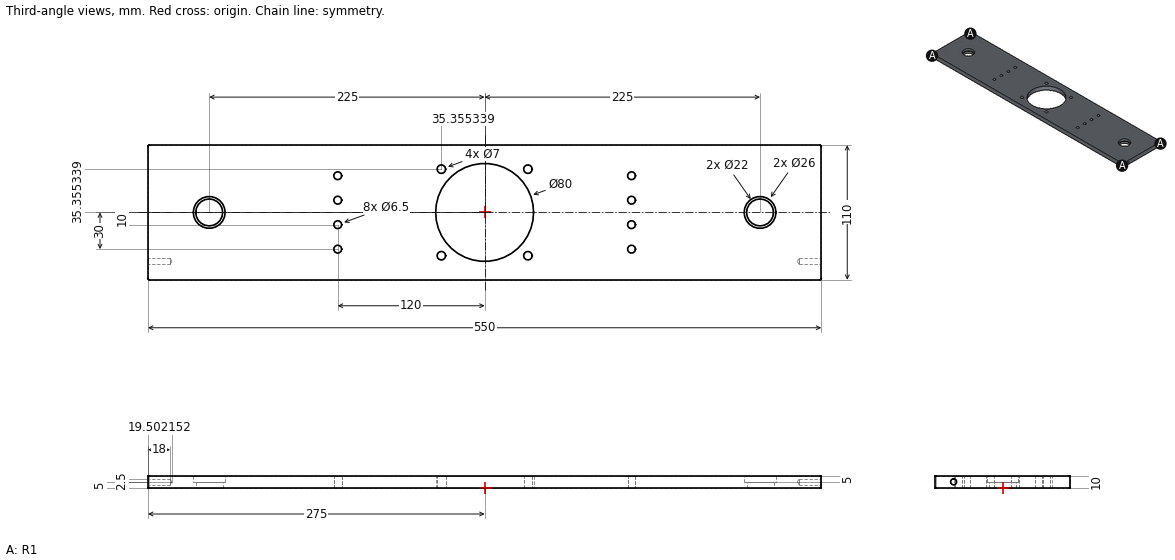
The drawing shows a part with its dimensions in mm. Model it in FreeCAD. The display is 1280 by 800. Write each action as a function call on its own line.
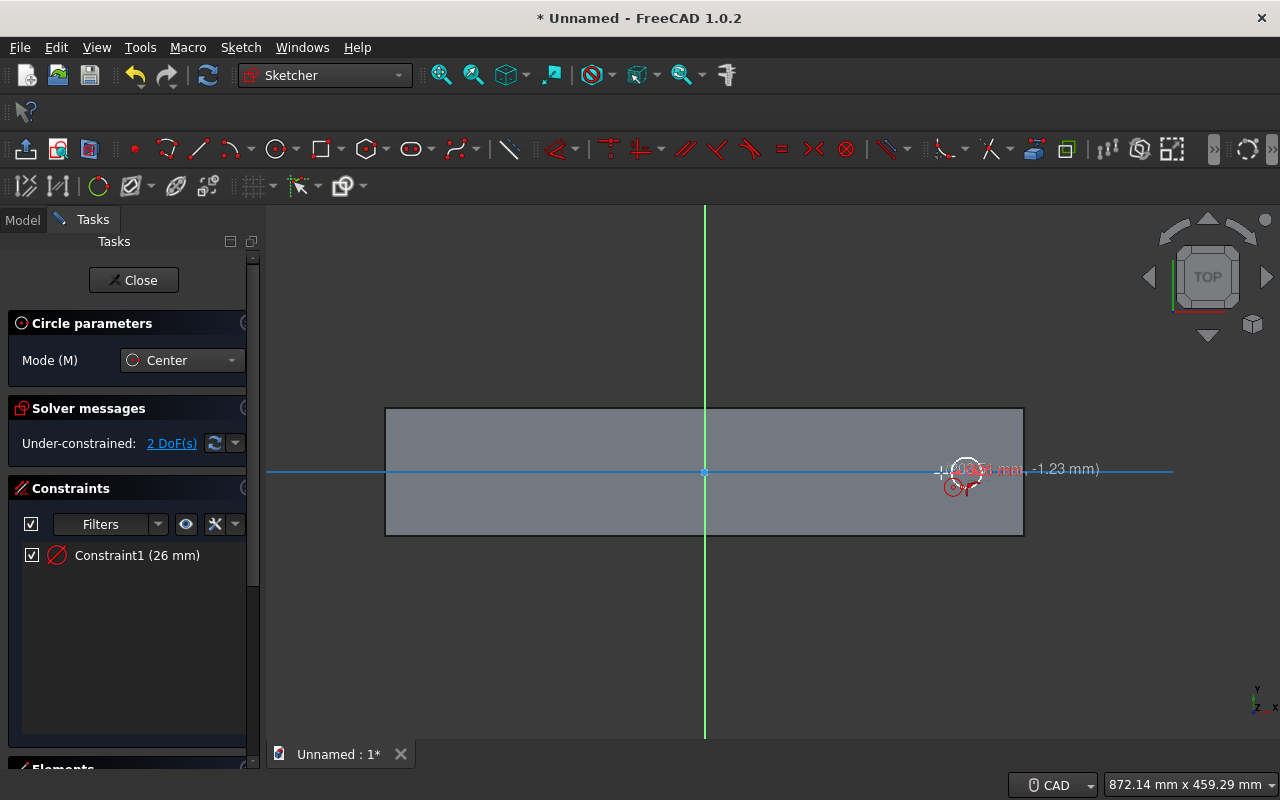
scroll(443, 472, up, 3)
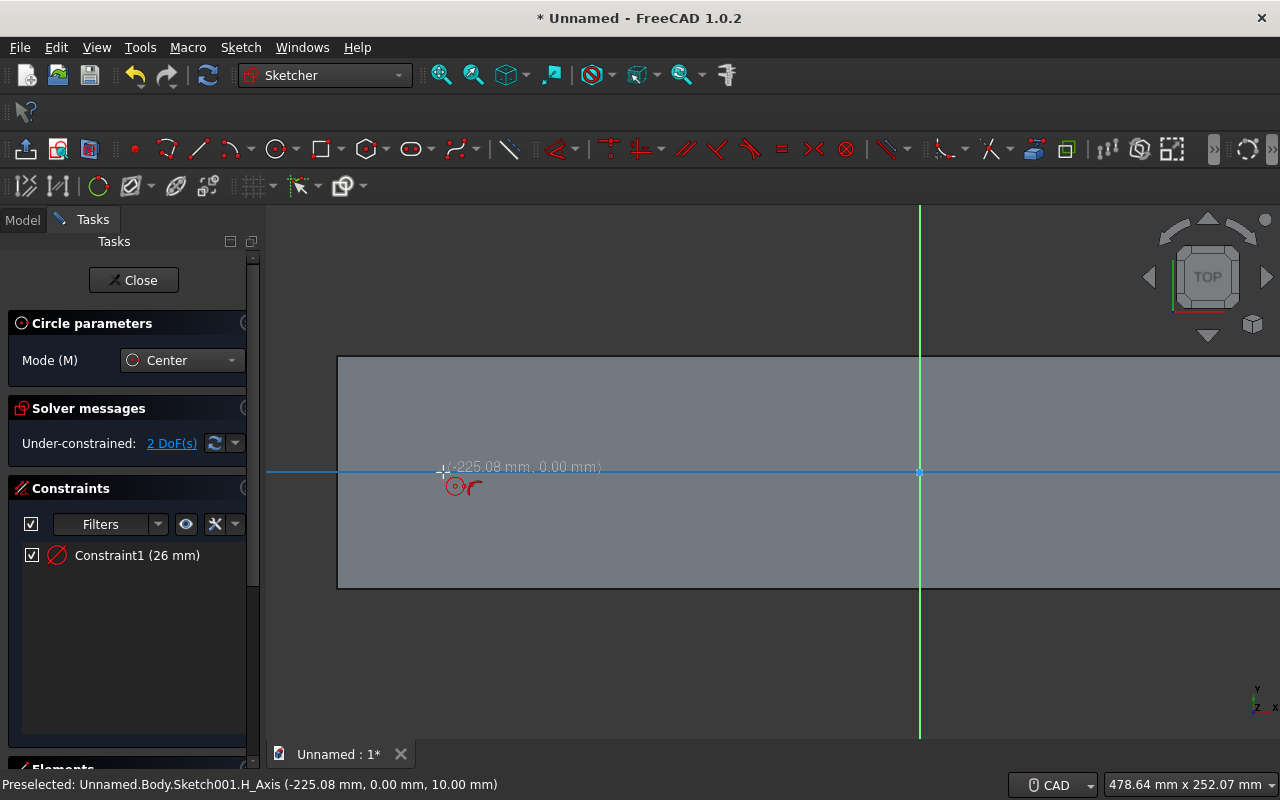
click(443, 472)
move(462, 453)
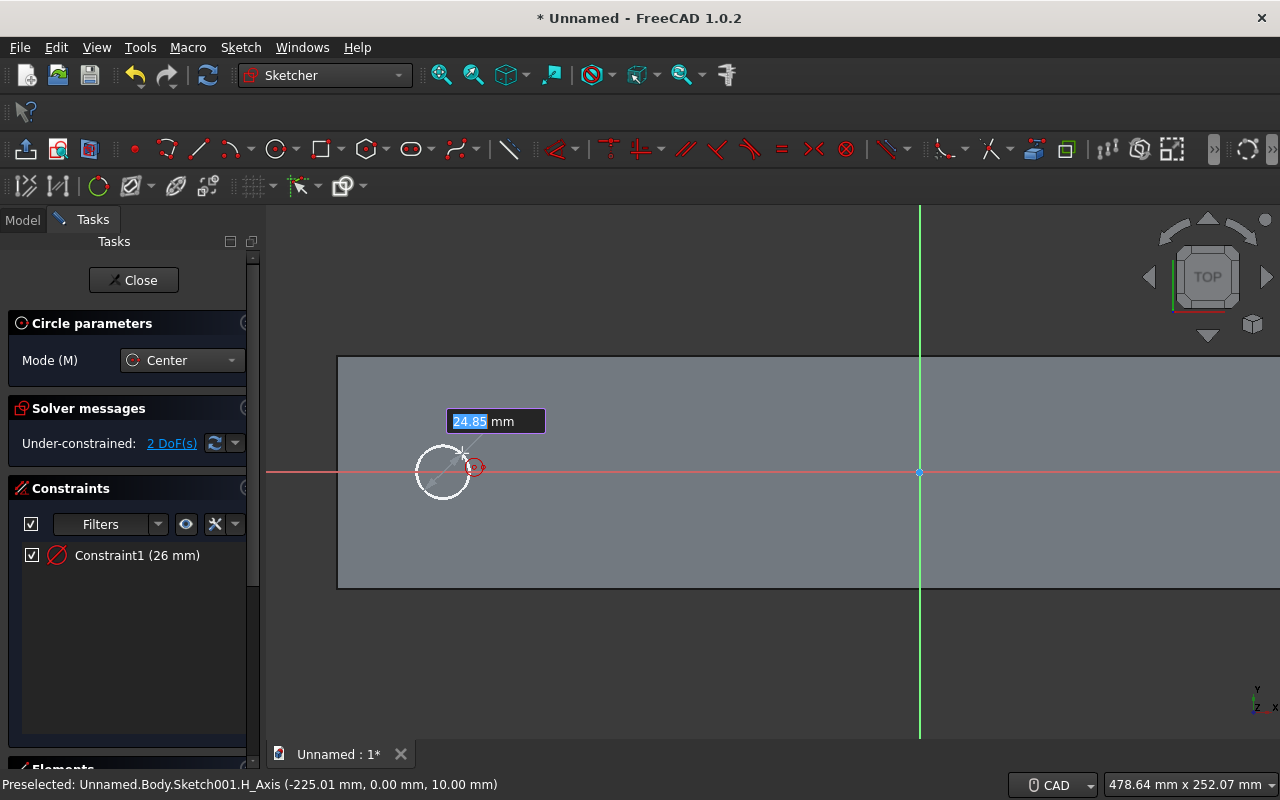
text(26)
key(Return)
key(Escape)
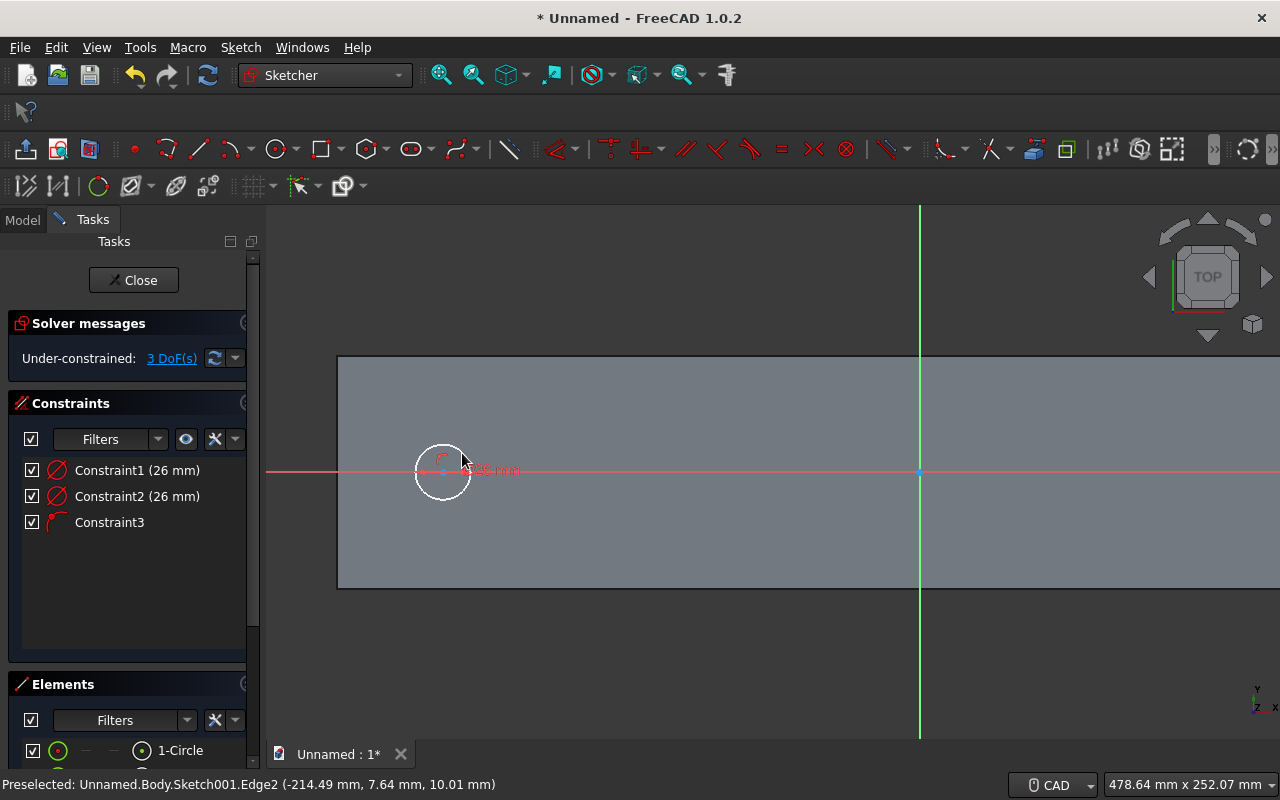
scroll(443, 472, down, 3)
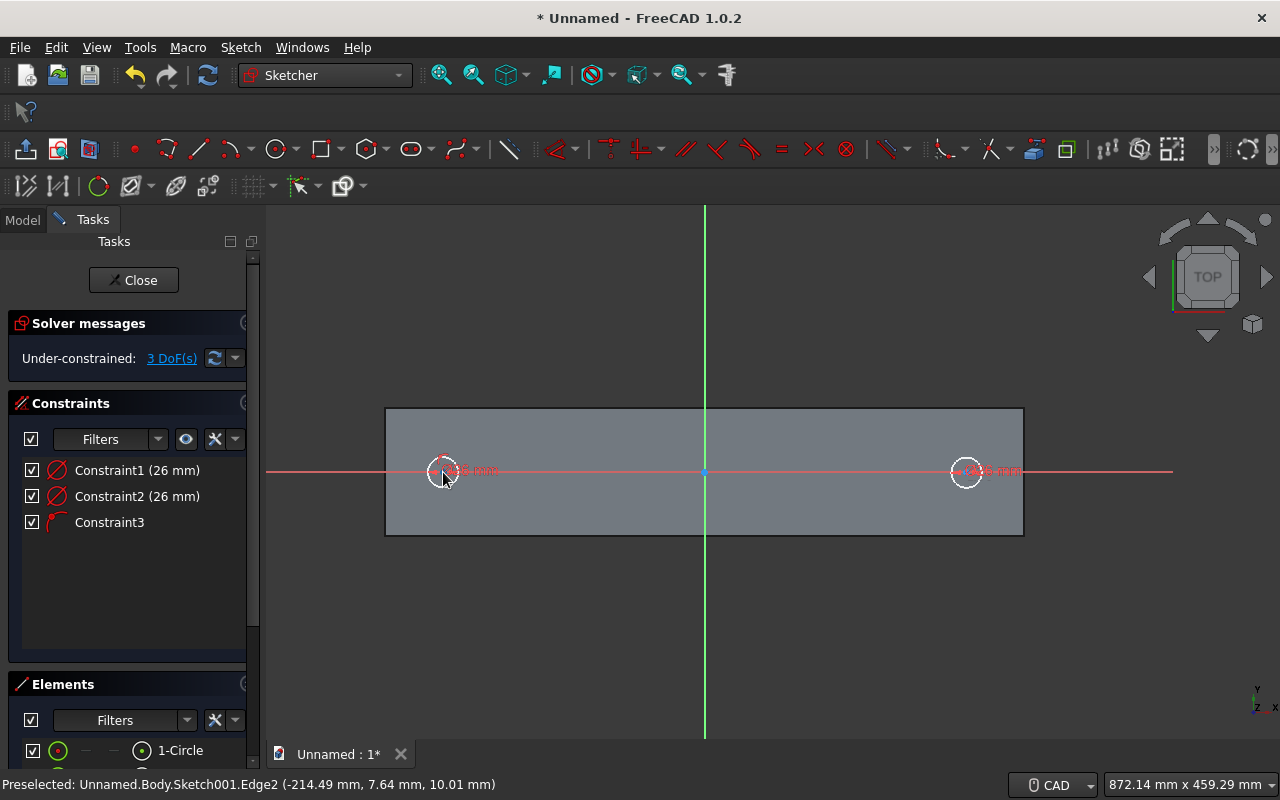
click(967, 473)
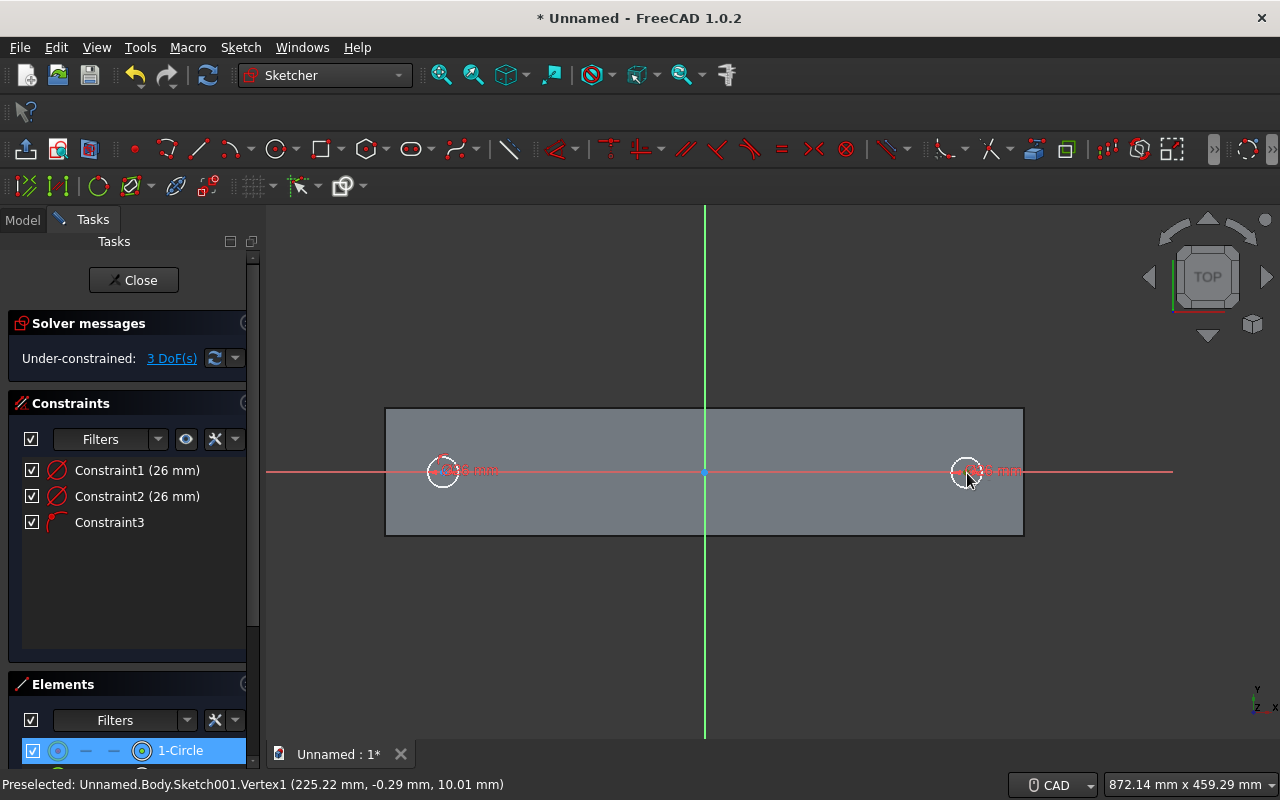
click(353, 472)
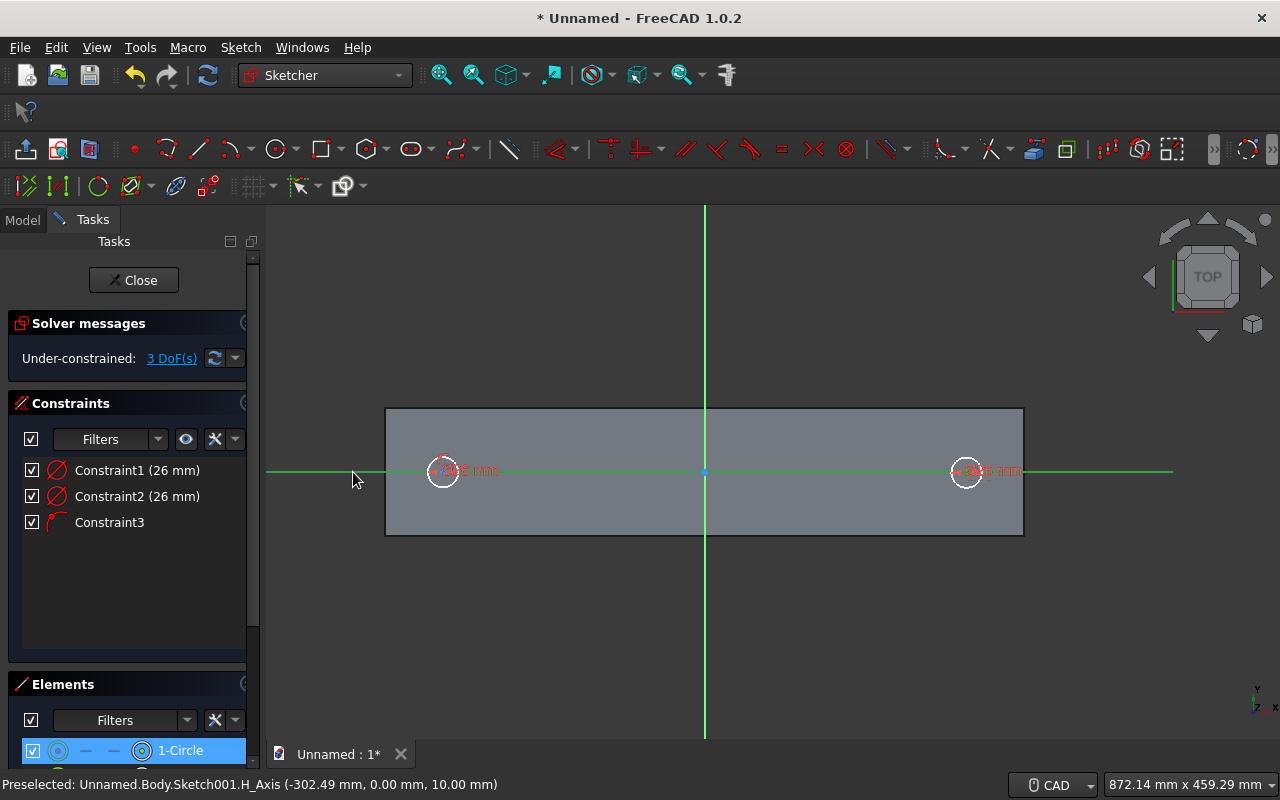
key(c)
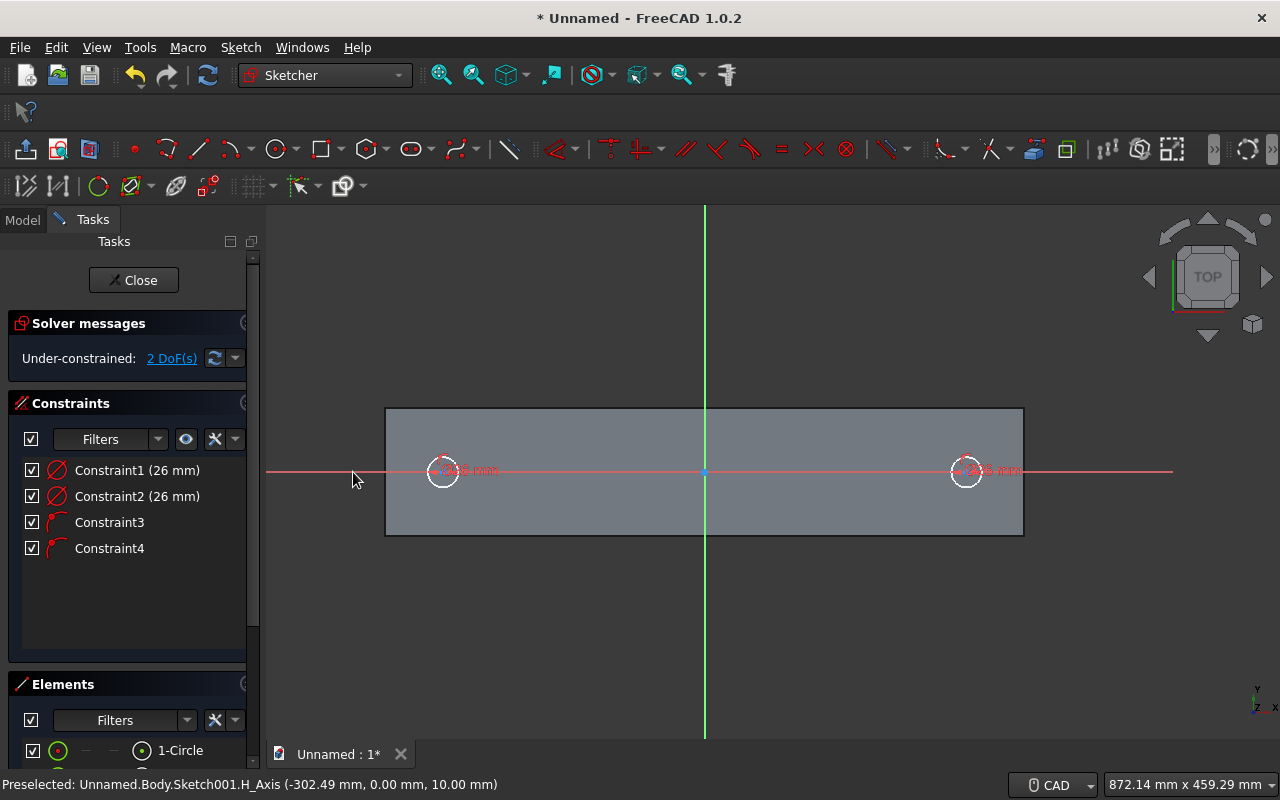
click(967, 472)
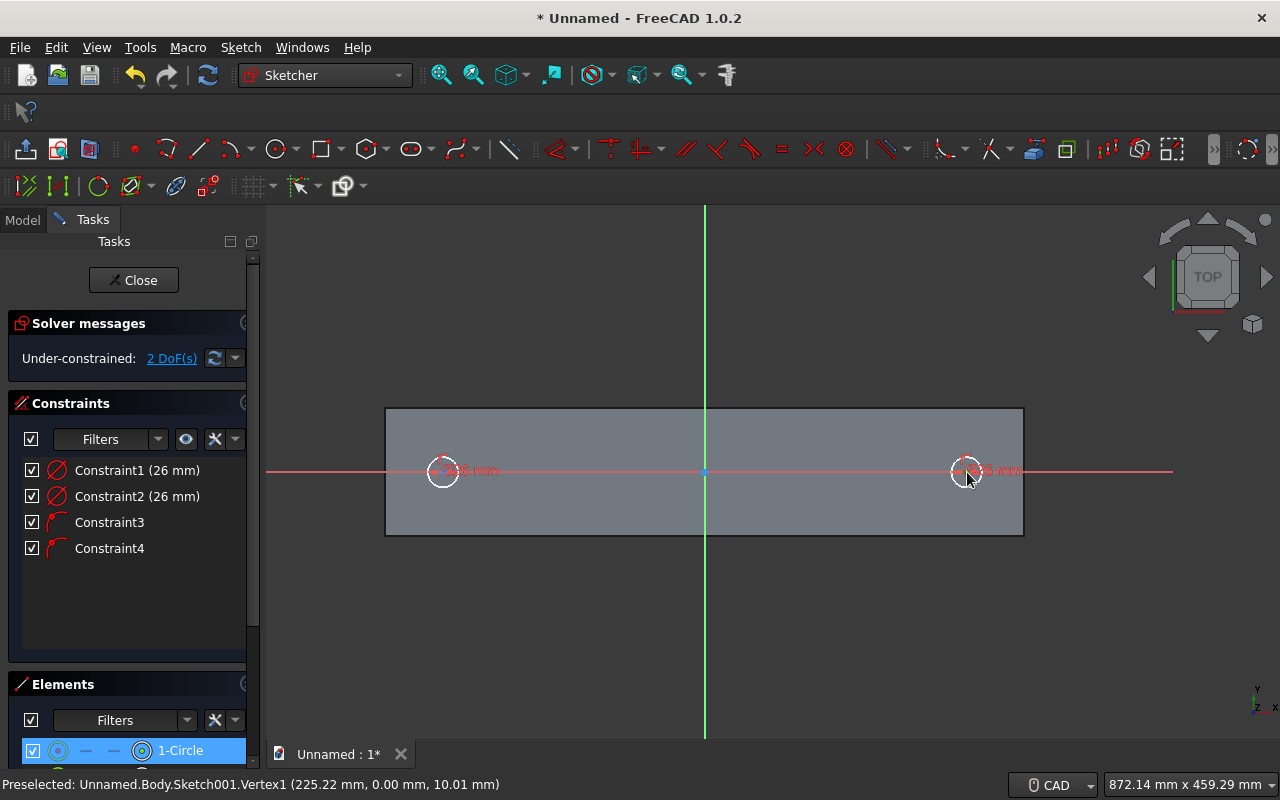
click(578, 150)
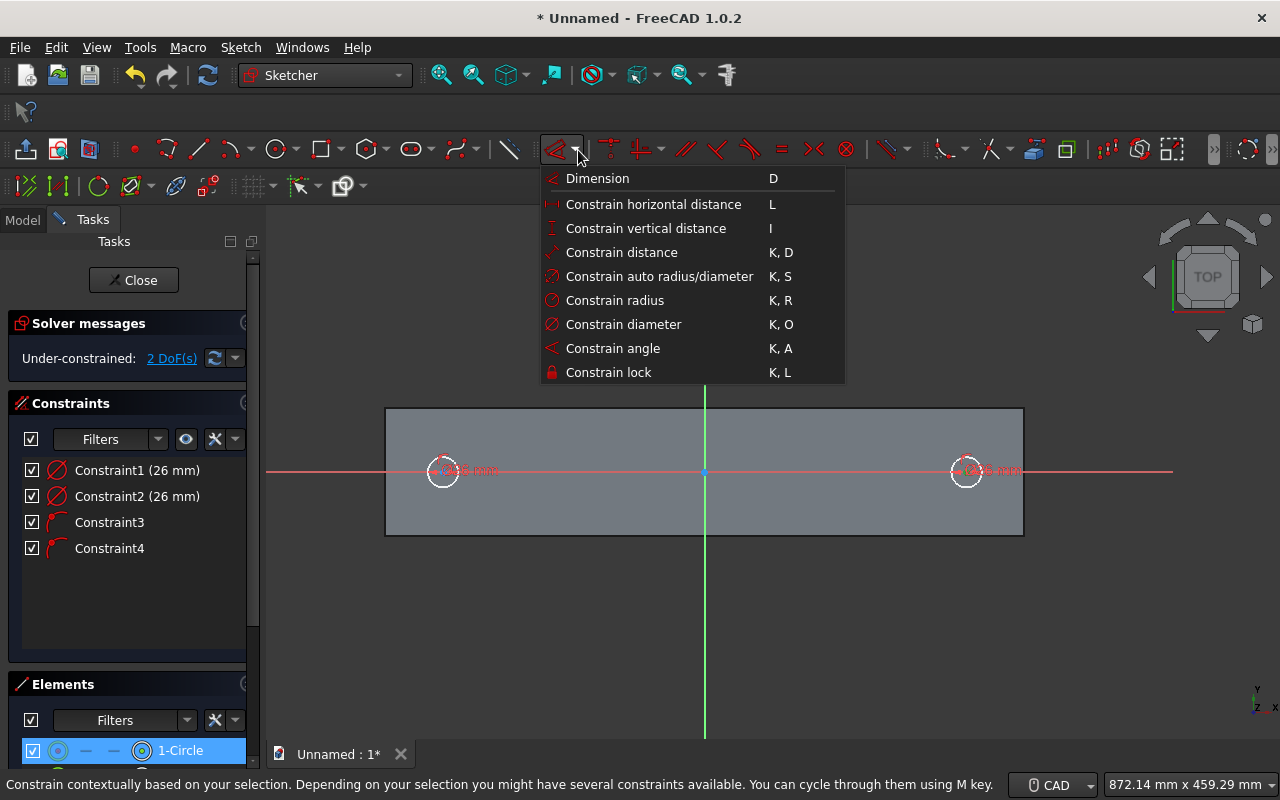
click(693, 204)